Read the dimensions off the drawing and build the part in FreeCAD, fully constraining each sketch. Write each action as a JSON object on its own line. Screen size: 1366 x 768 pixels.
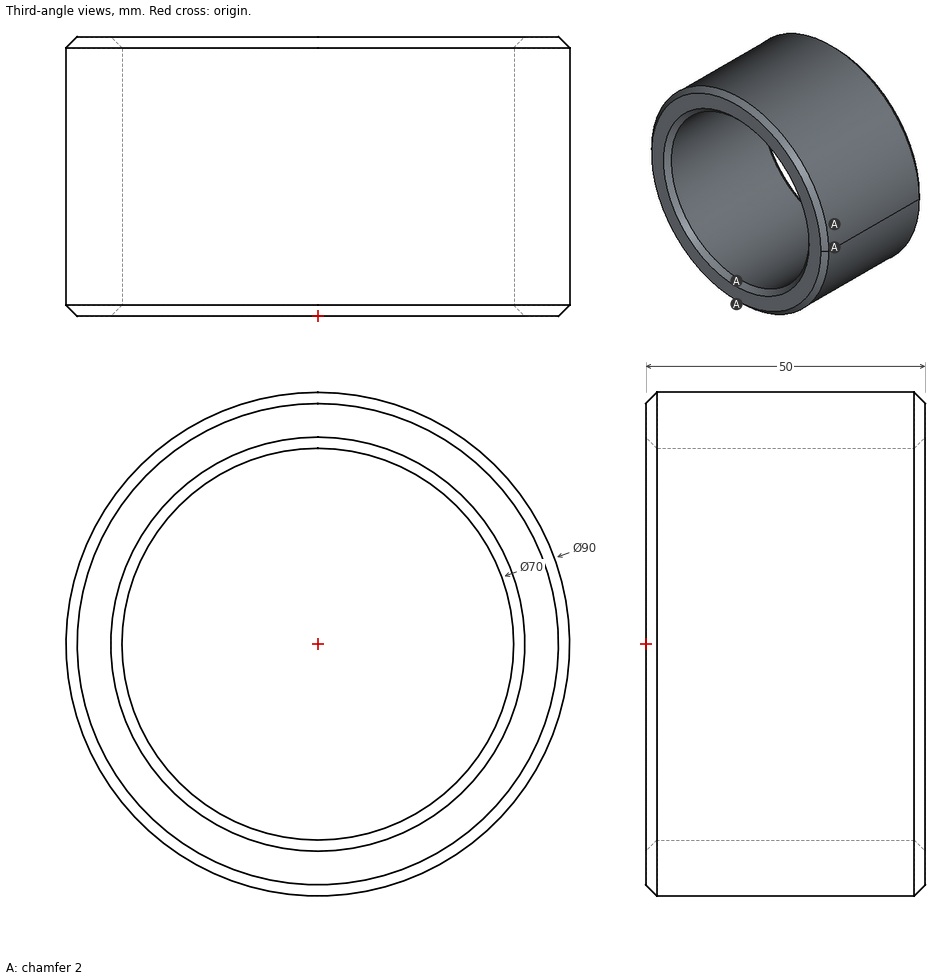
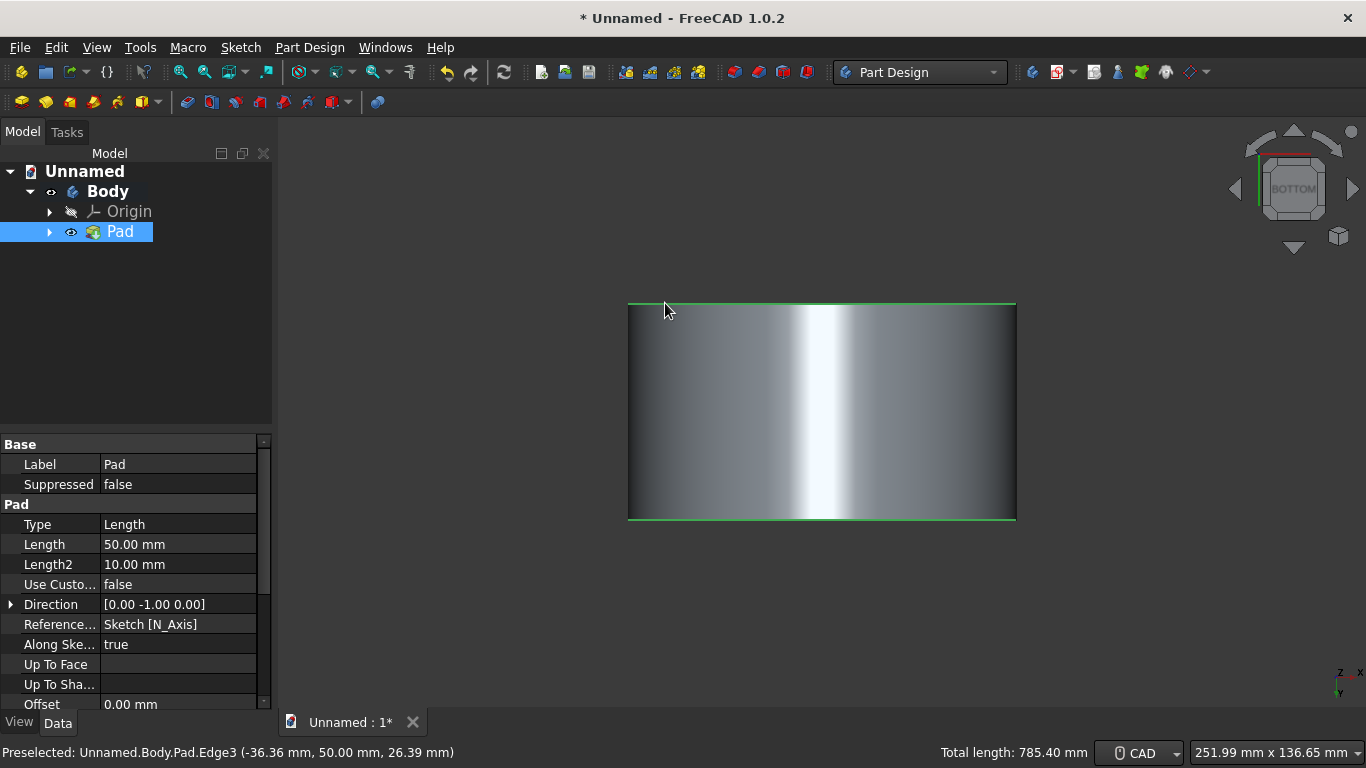
{"action": "left_click", "coordinate": [182, 72]}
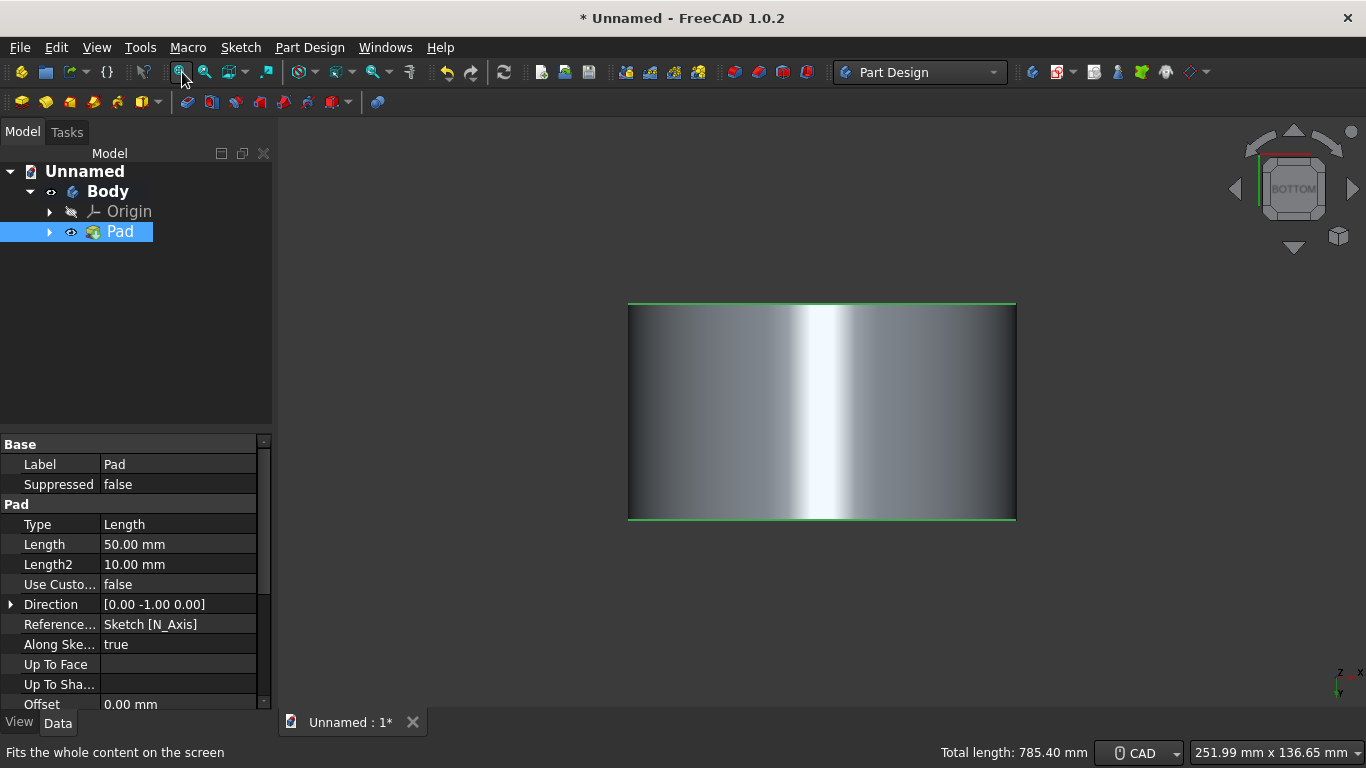
{"action": "key", "text": "4"}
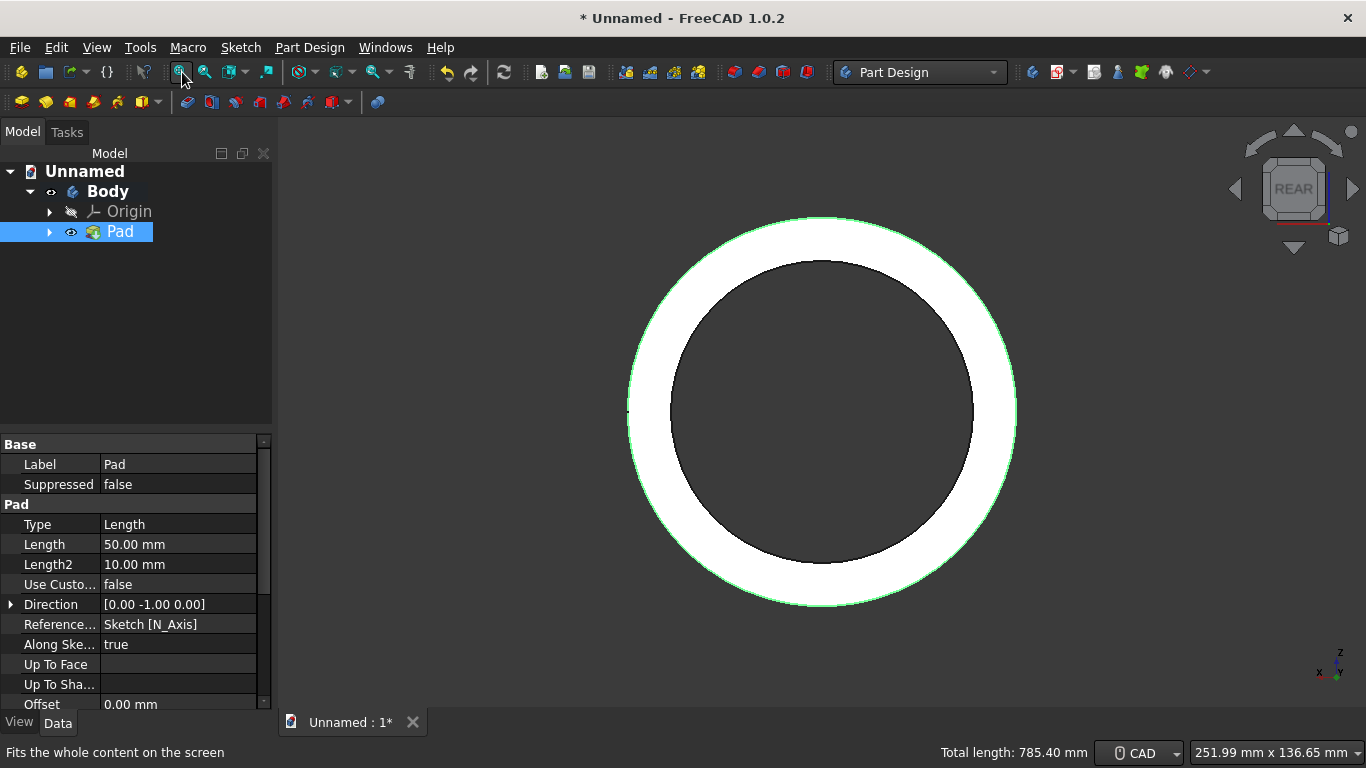
{"action": "left_click", "coordinate": [944, 322], "text": "ctrl"}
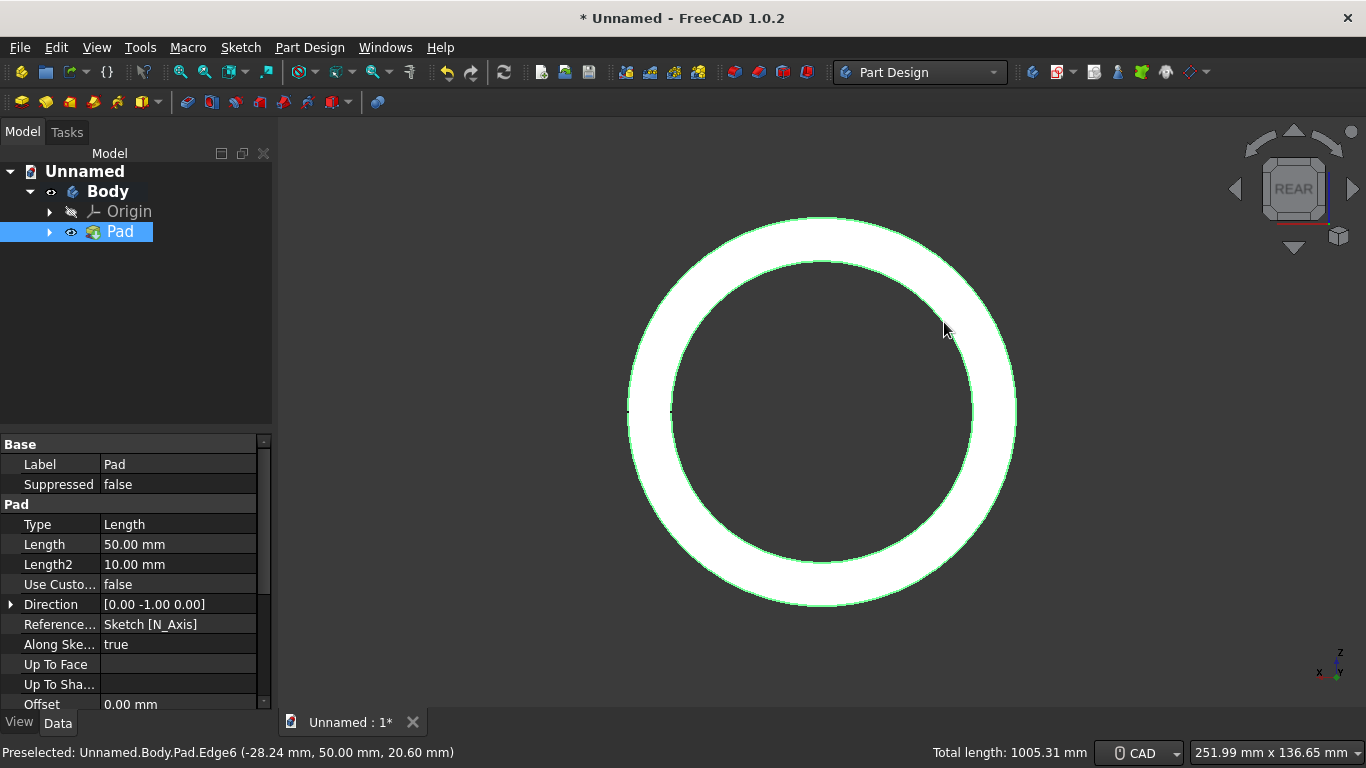
{"action": "left_click", "coordinate": [760, 72]}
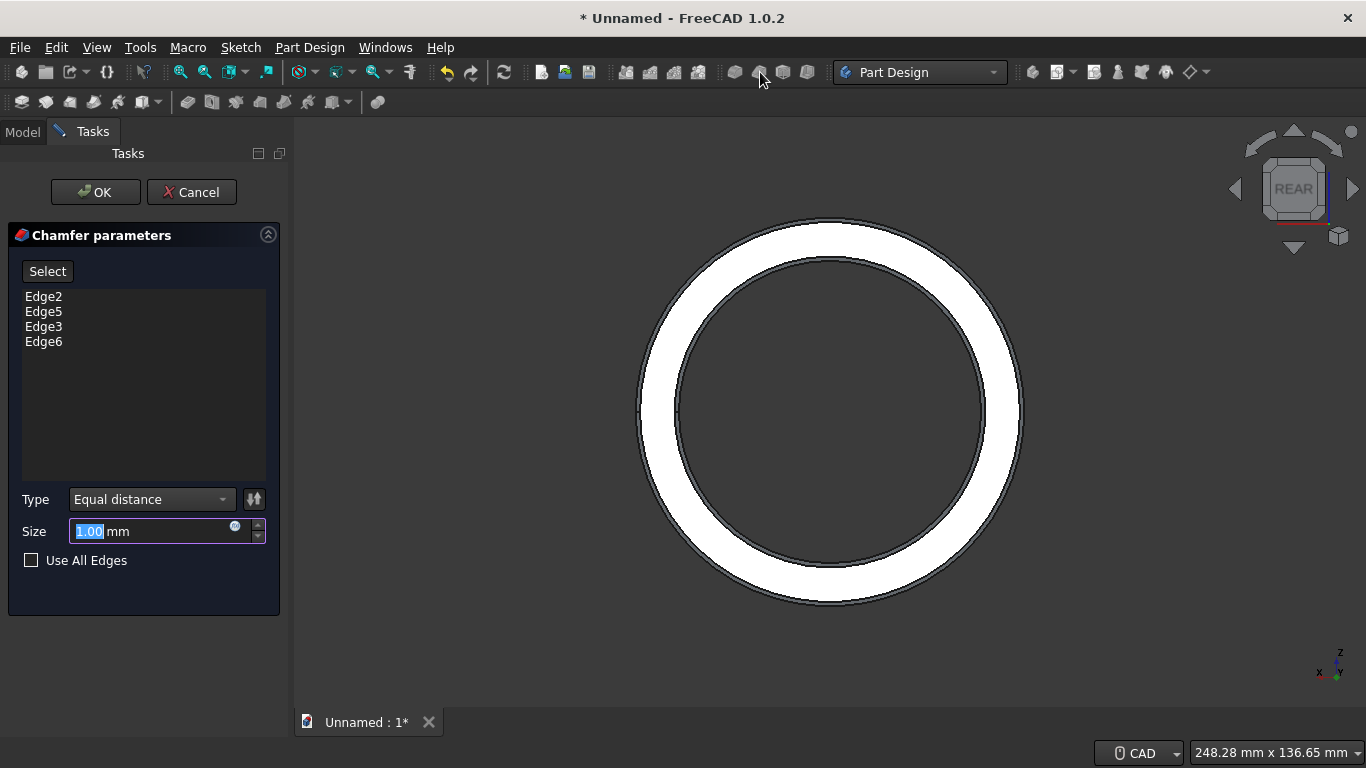
{"action": "type", "text": "2"}
{"action": "key", "text": "Tab"}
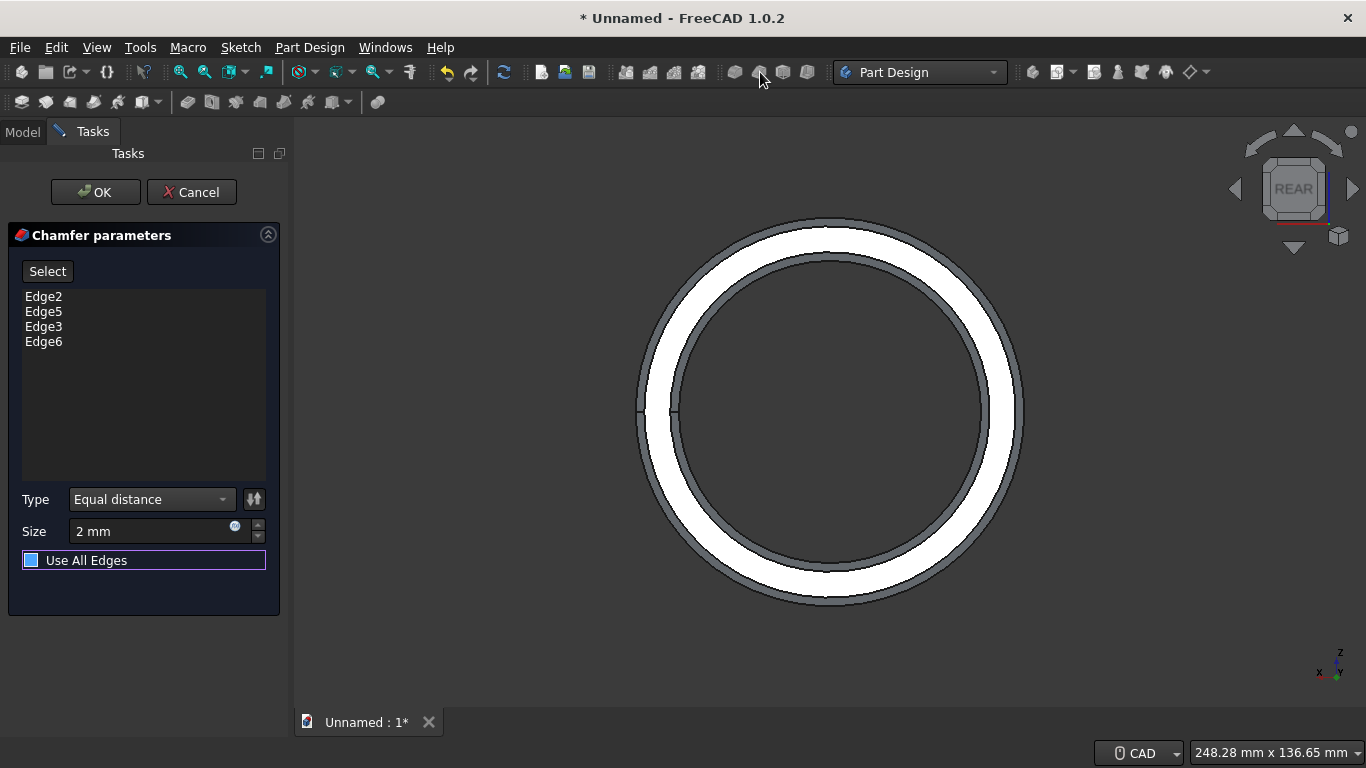
{"action": "left_click", "coordinate": [96, 192]}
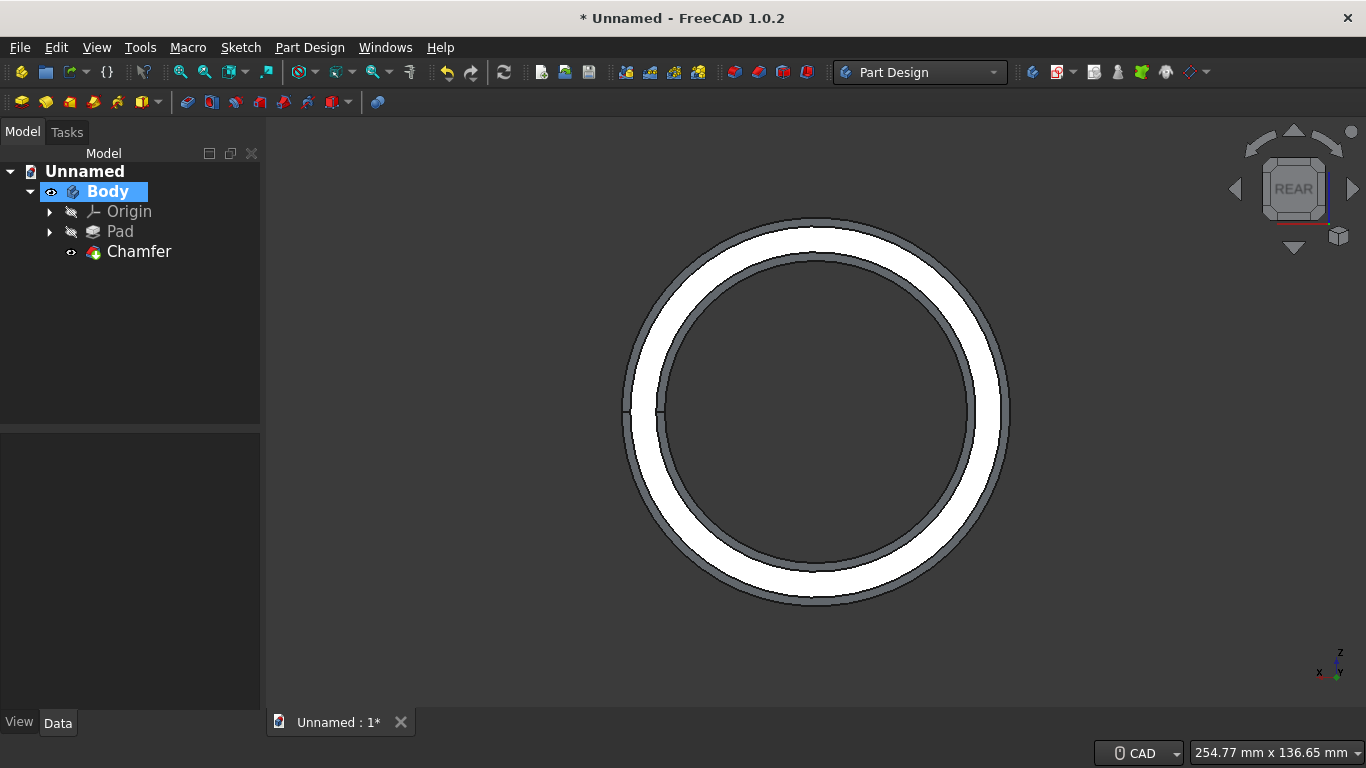
{"action": "key", "text": "0"}